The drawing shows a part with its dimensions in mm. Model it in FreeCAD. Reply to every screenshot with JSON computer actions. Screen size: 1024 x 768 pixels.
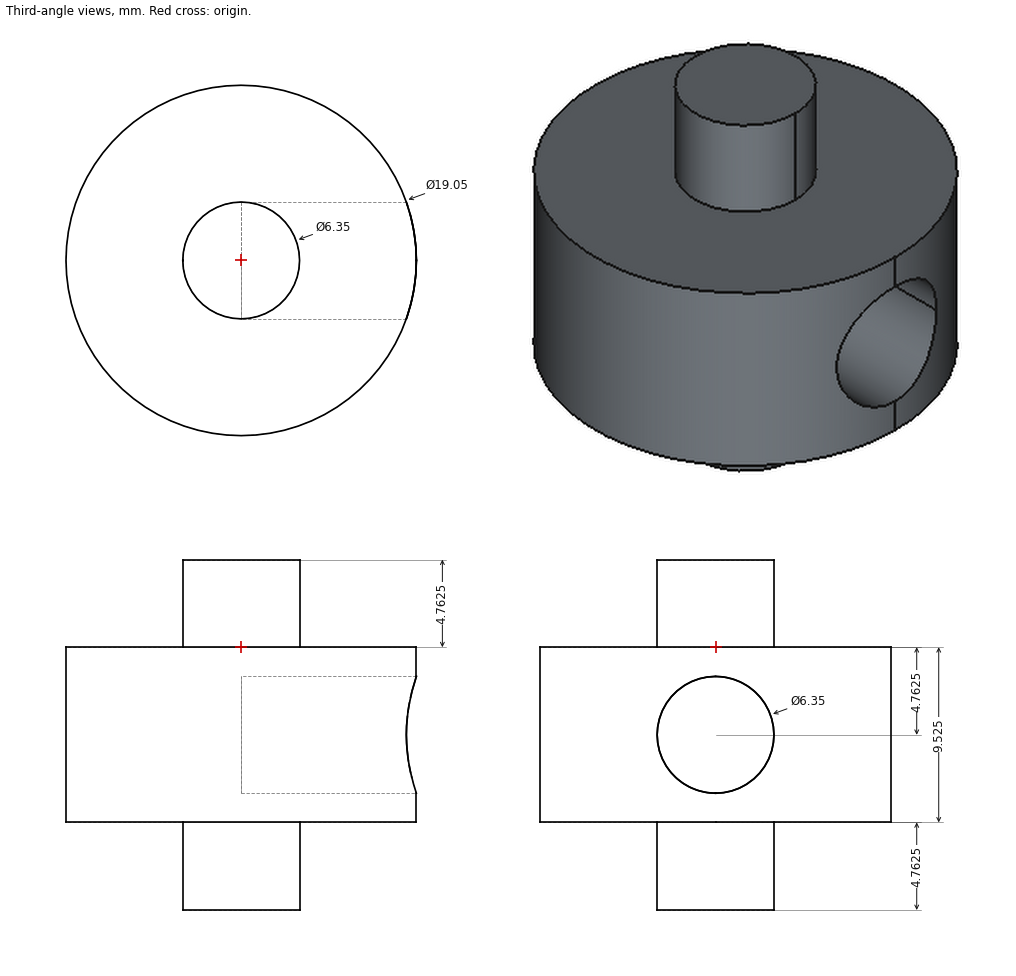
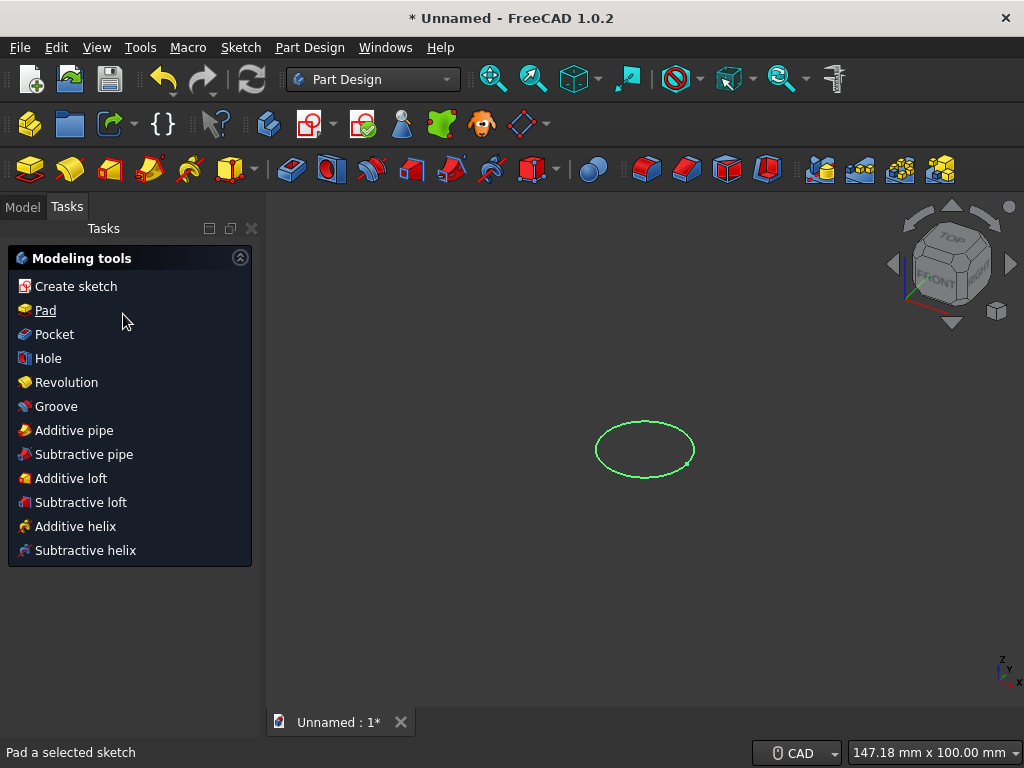
{"action": "left_click", "coordinate": [30, 170]}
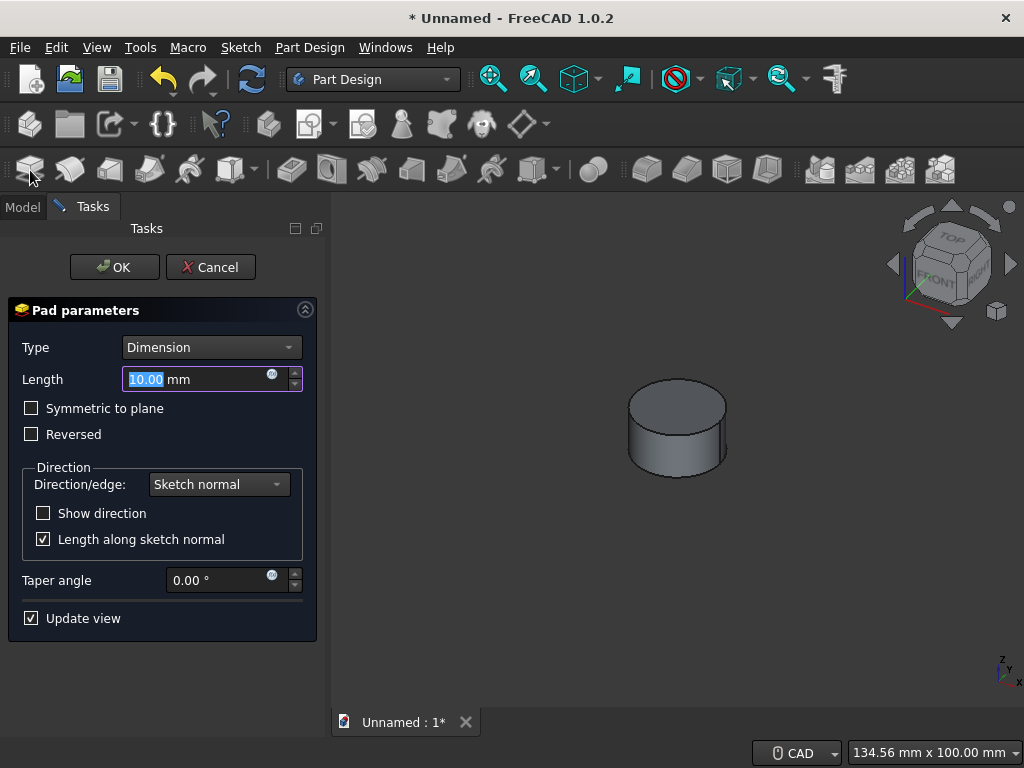
{"action": "type", "text": "9.525"}
{"action": "key", "text": "Tab"}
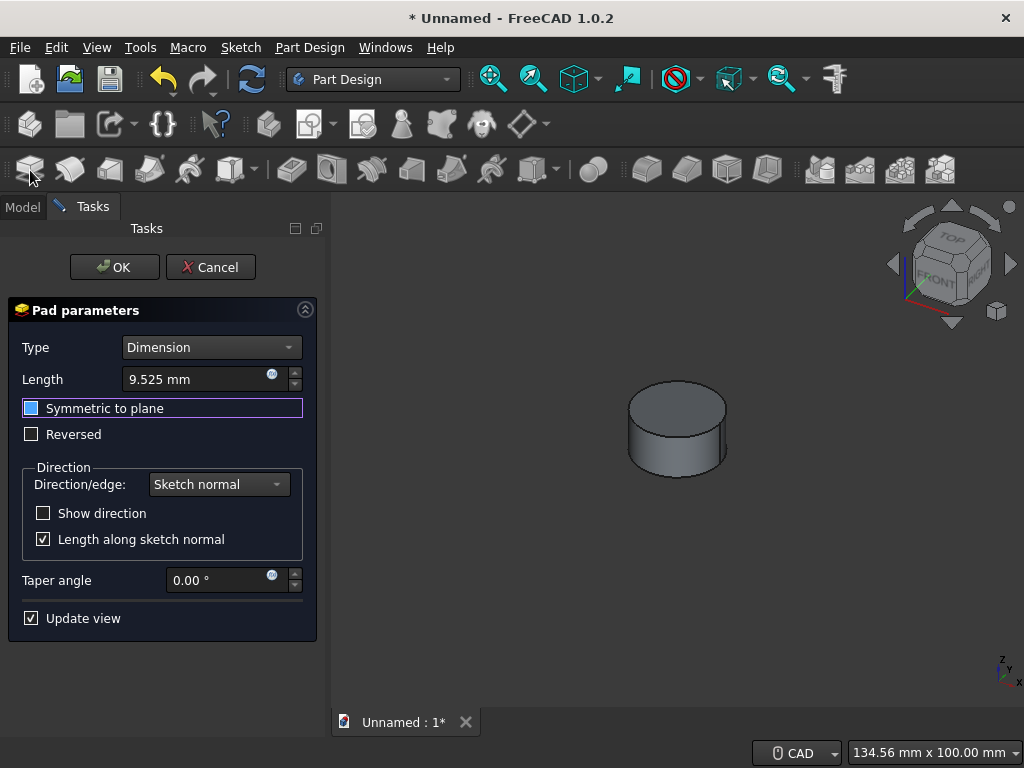
{"action": "left_click", "coordinate": [30, 434]}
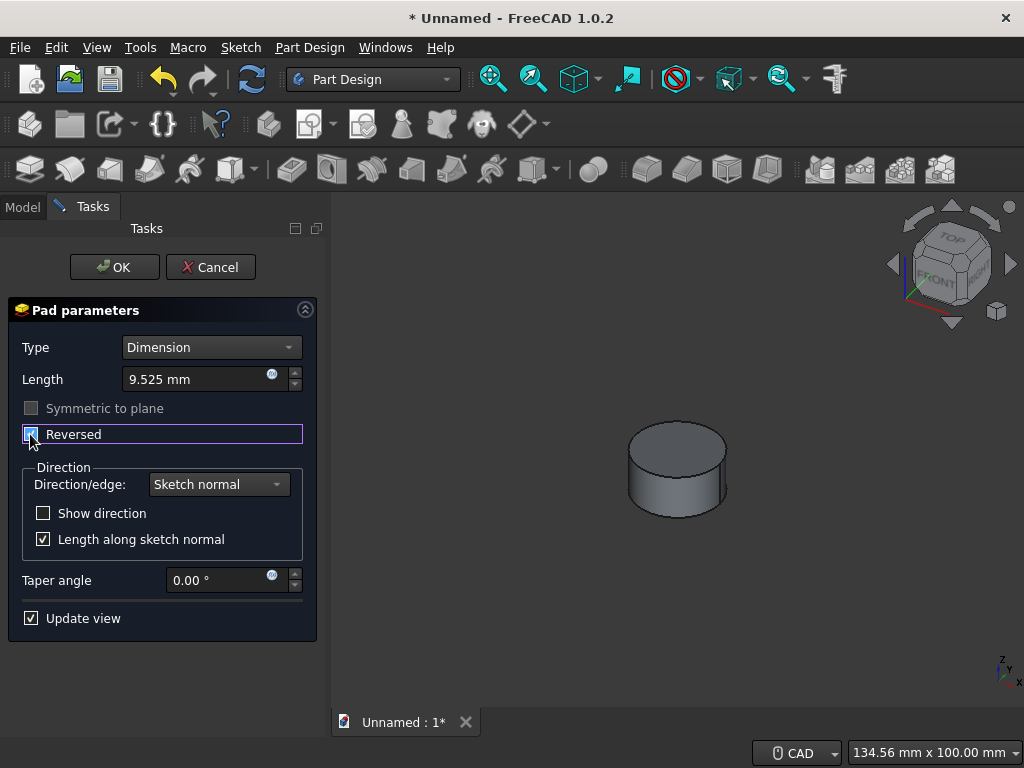
{"action": "left_click", "coordinate": [115, 267]}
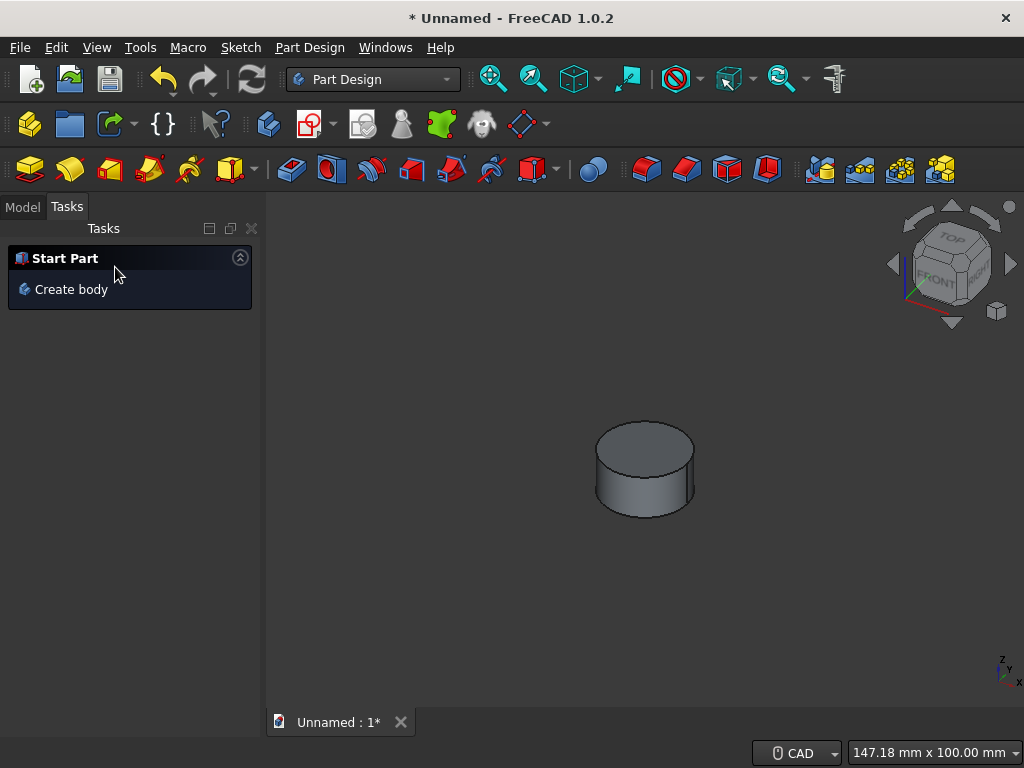
{"action": "key", "text": "v f"}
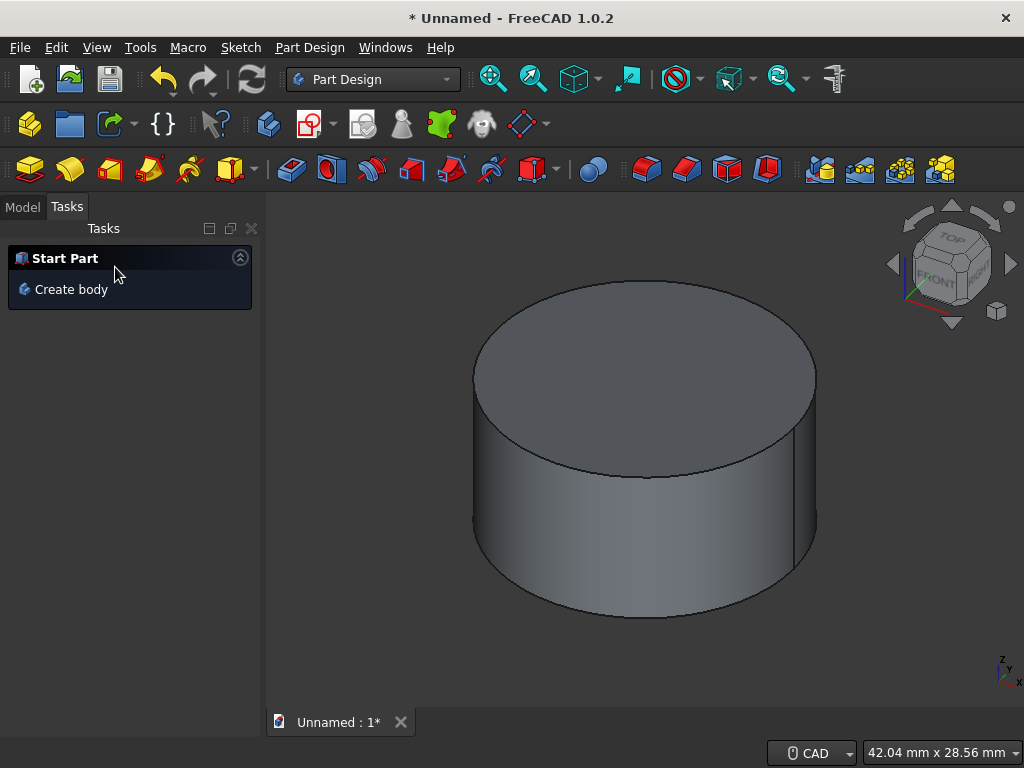
{"action": "left_click", "coordinate": [310, 124]}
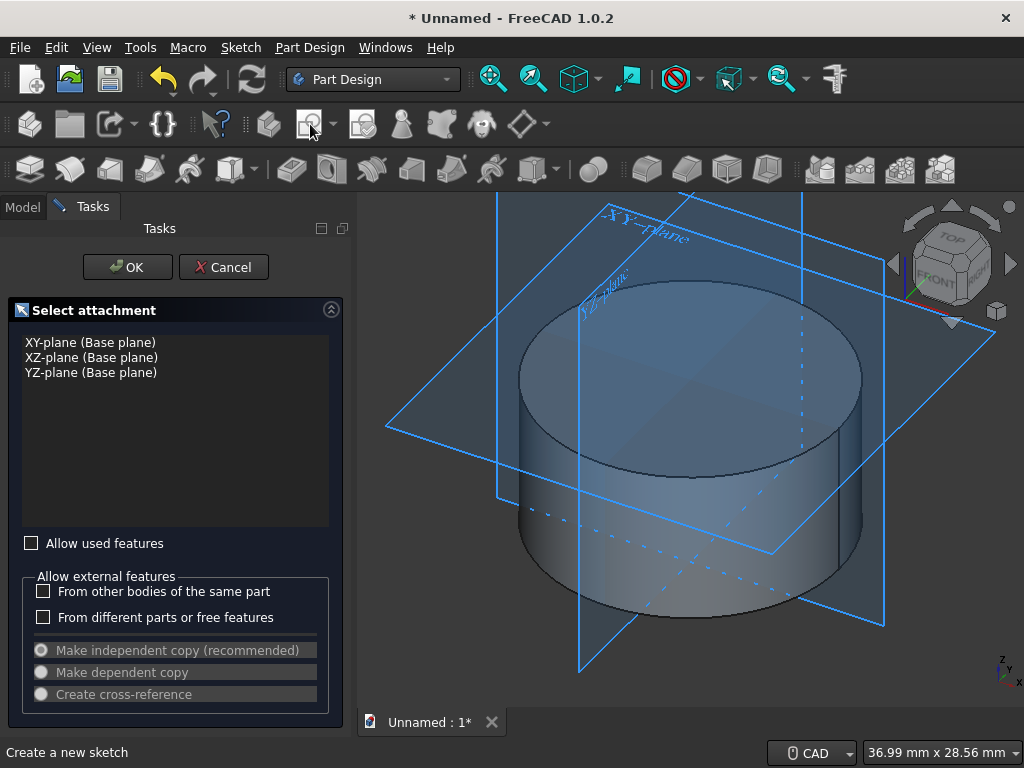
{"action": "left_click", "coordinate": [82, 342]}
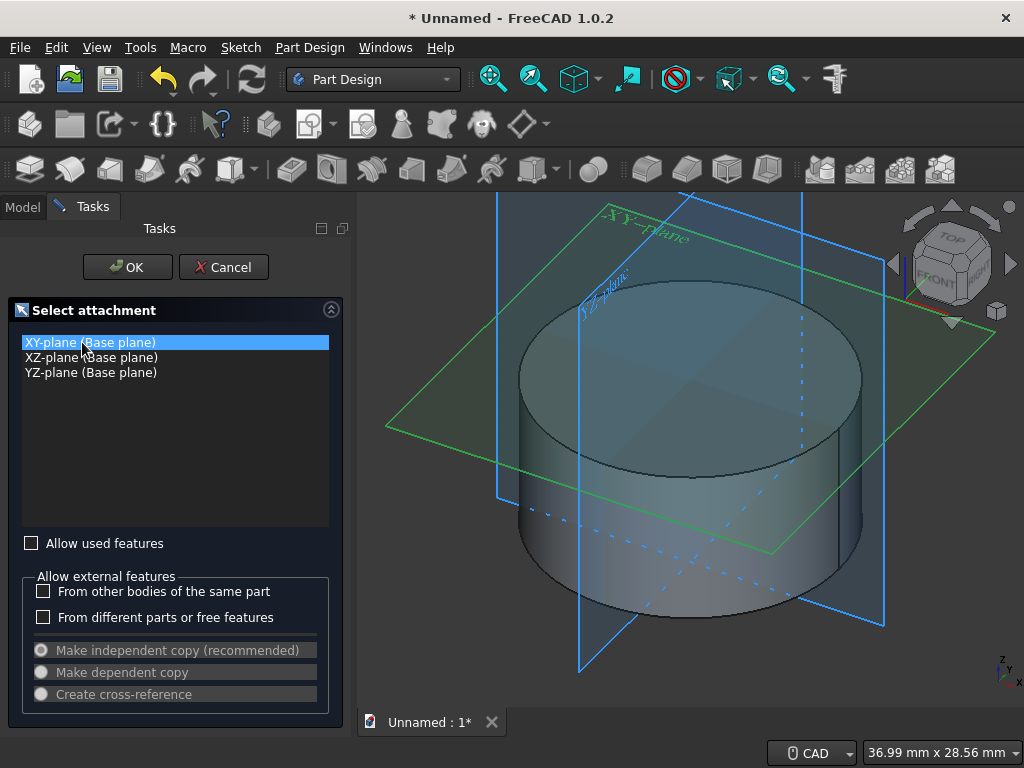
{"action": "left_click", "coordinate": [128, 267]}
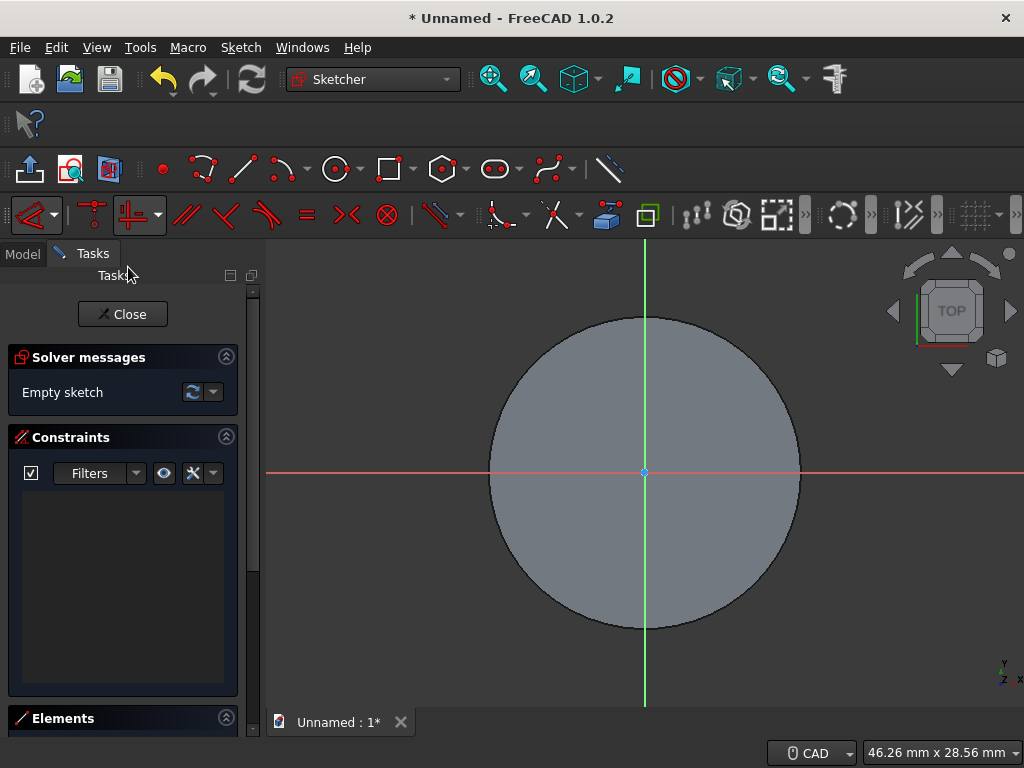
{"action": "scroll", "coordinate": [685, 473], "scroll_direction": "up", "scroll_amount": 5}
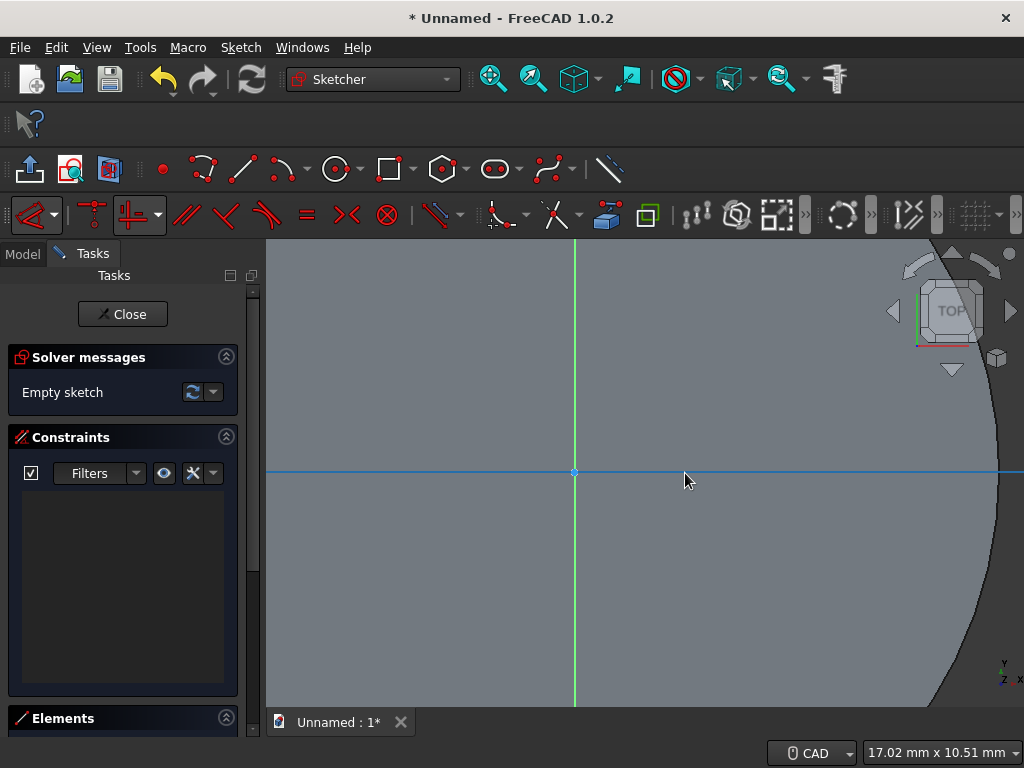
{"action": "key", "text": "g c"}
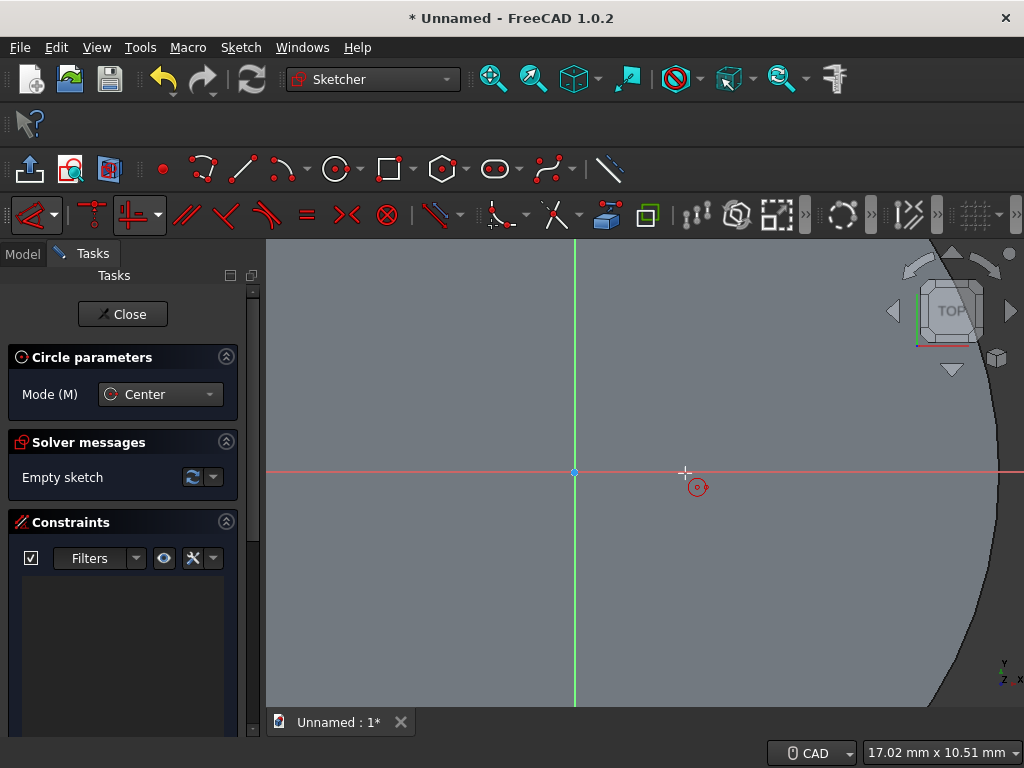
{"action": "left_click", "coordinate": [575, 472]}
{"action": "left_click", "coordinate": [675, 372]}
{"action": "key", "text": "Escape"}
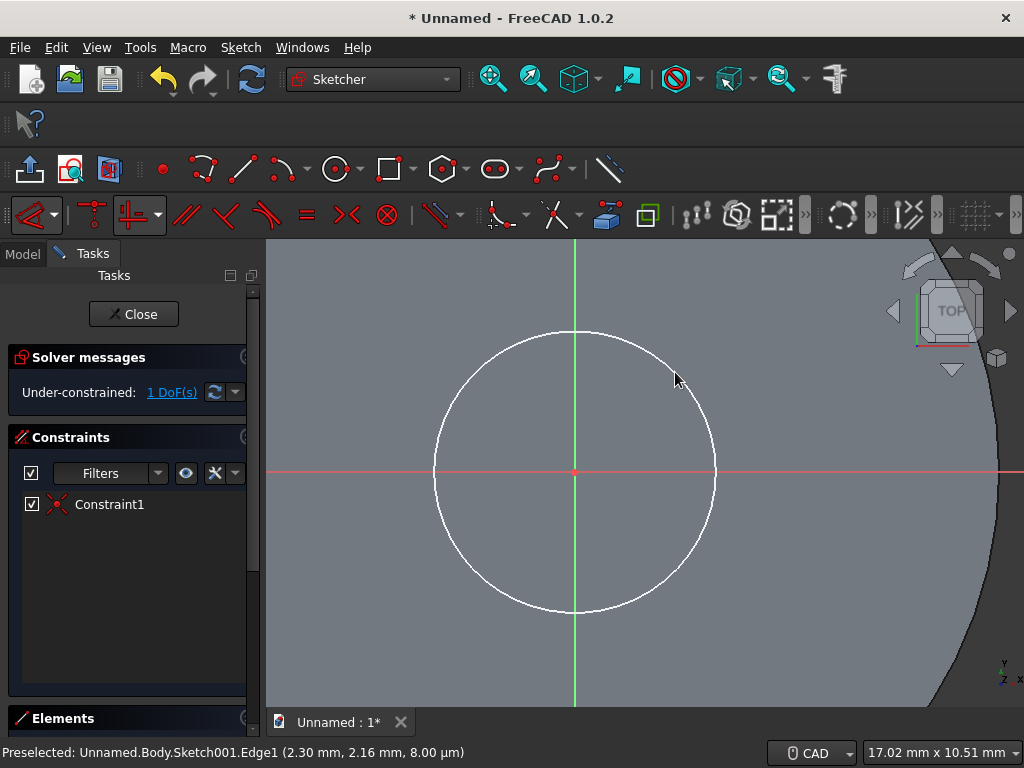
{"action": "left_click", "coordinate": [674, 372]}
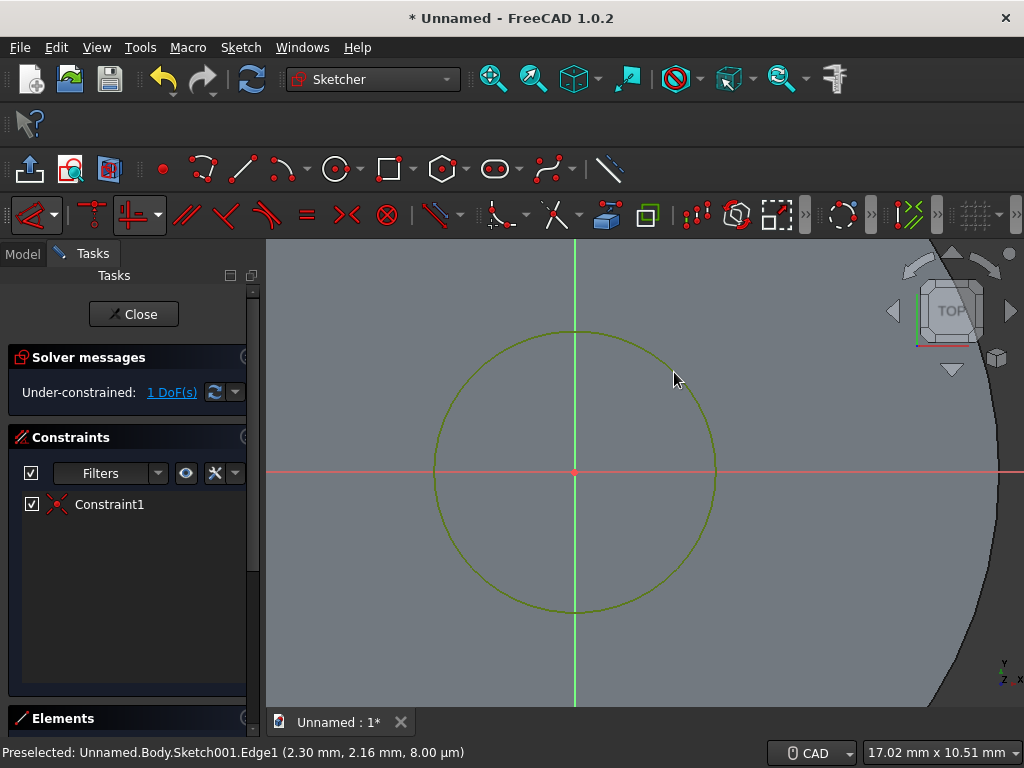
{"action": "key", "text": "k o"}